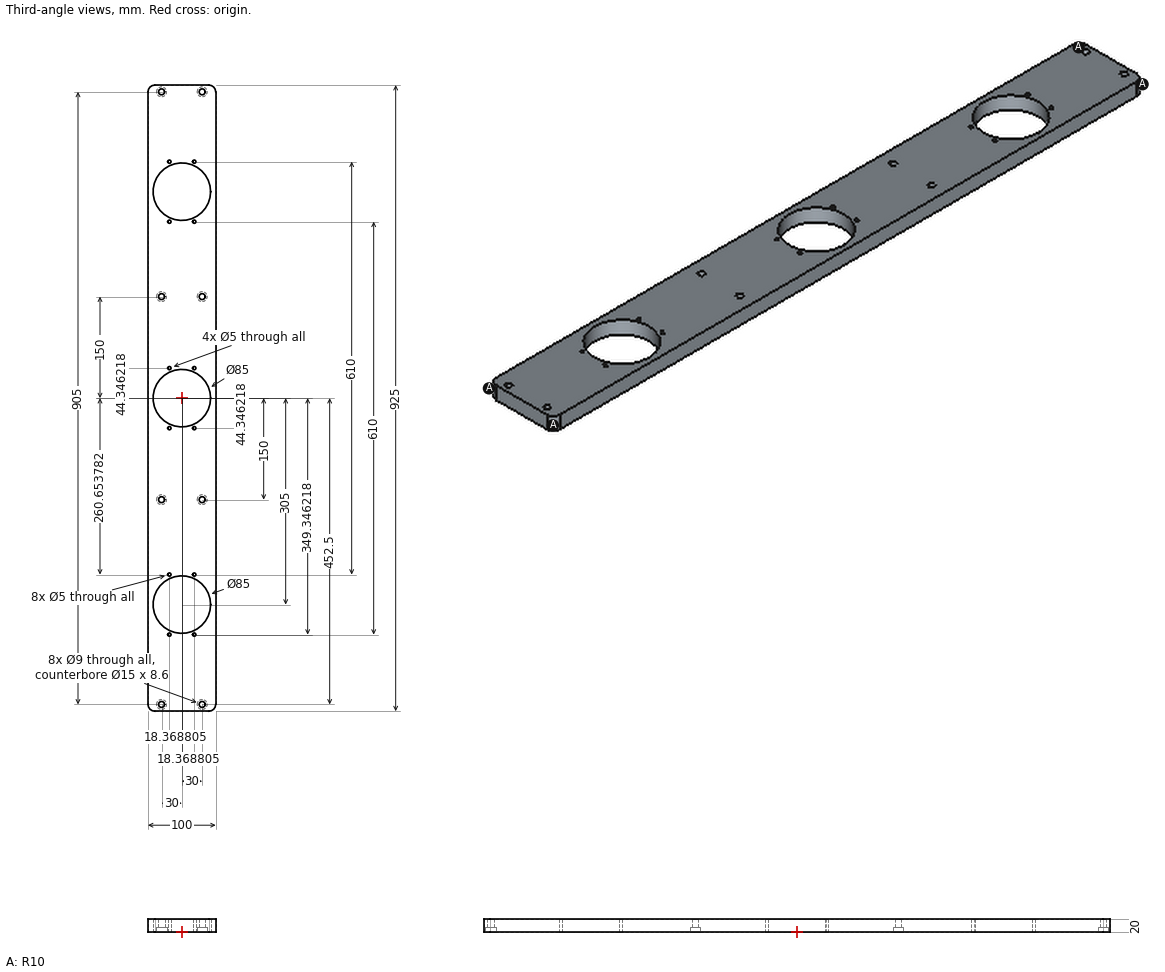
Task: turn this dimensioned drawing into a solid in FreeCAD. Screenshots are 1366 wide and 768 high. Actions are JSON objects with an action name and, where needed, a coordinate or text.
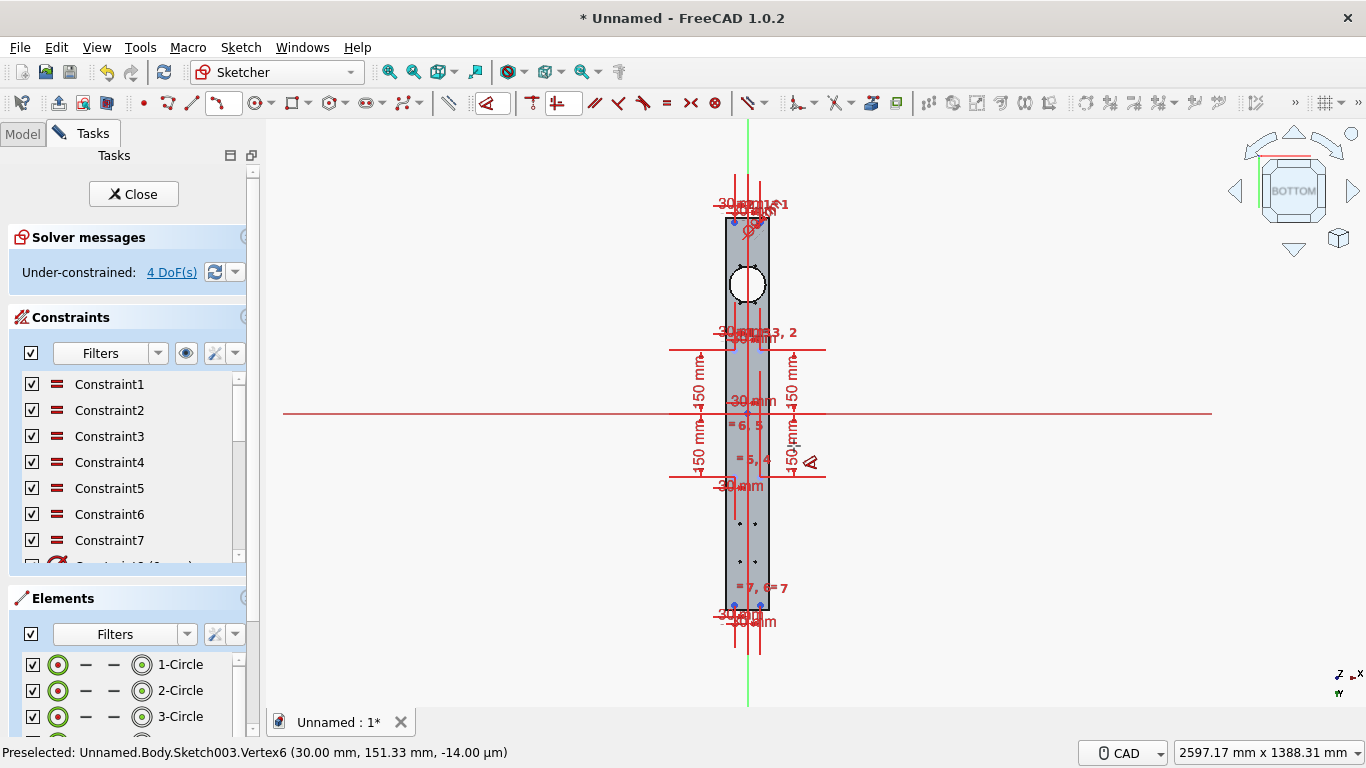
{"action": "left_click", "coordinate": [735, 223]}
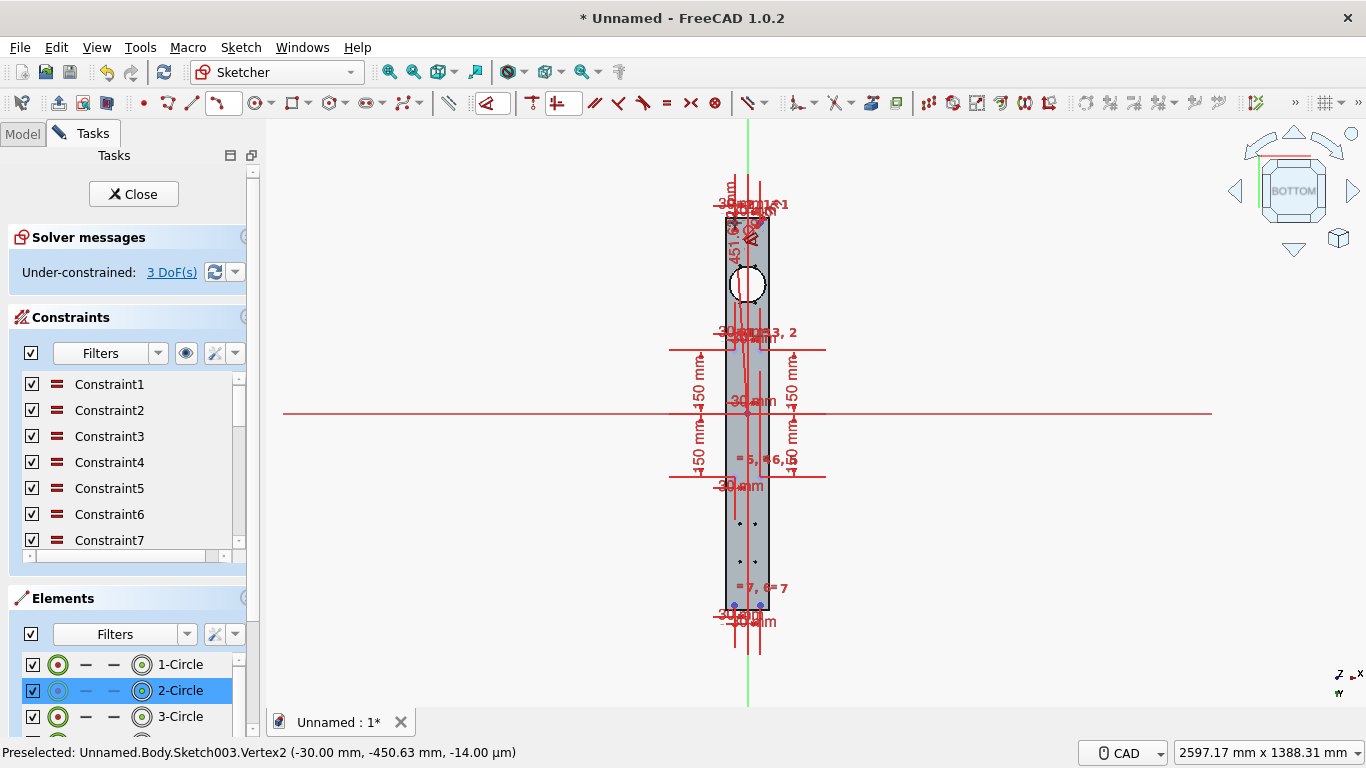
{"action": "left_click", "coordinate": [735, 606]}
{"action": "left_click", "coordinate": [701, 280]}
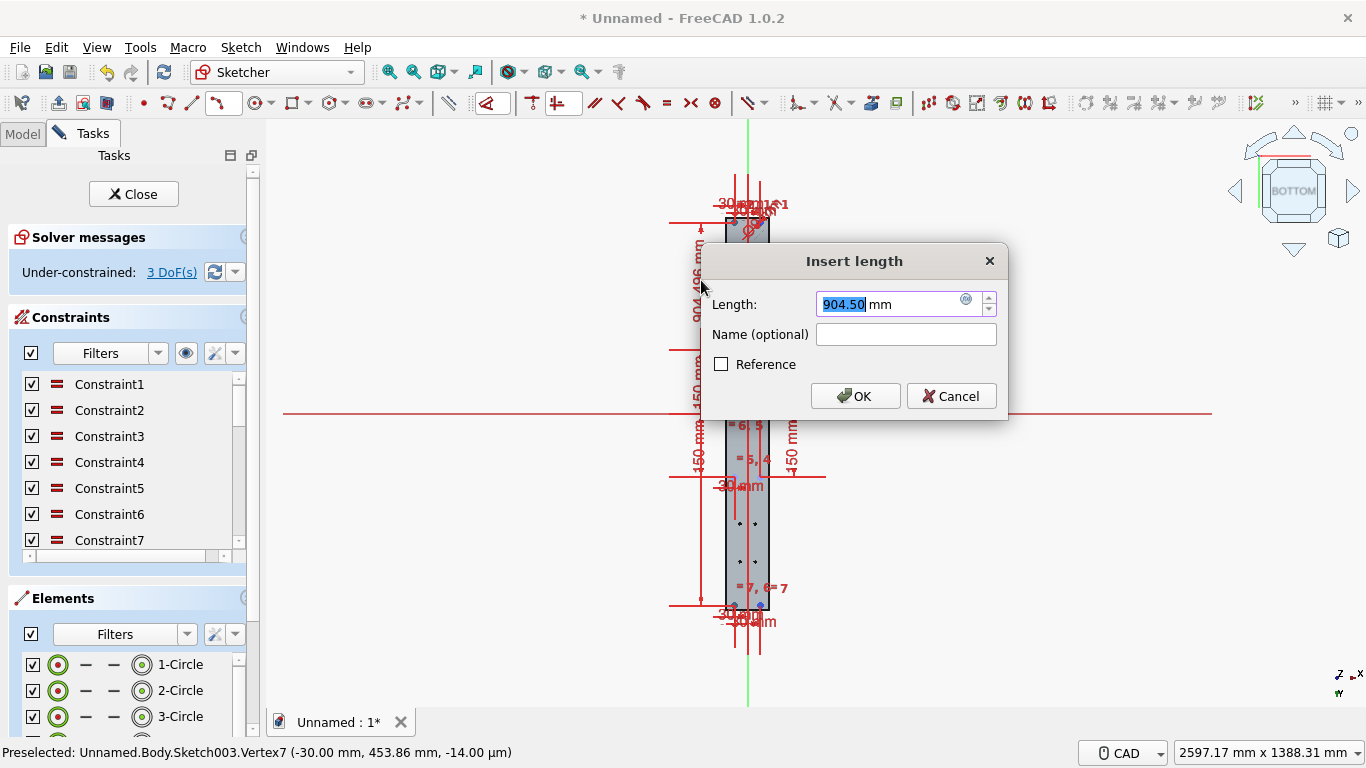
{"action": "type", "text": "905"}
{"action": "key", "text": "Return"}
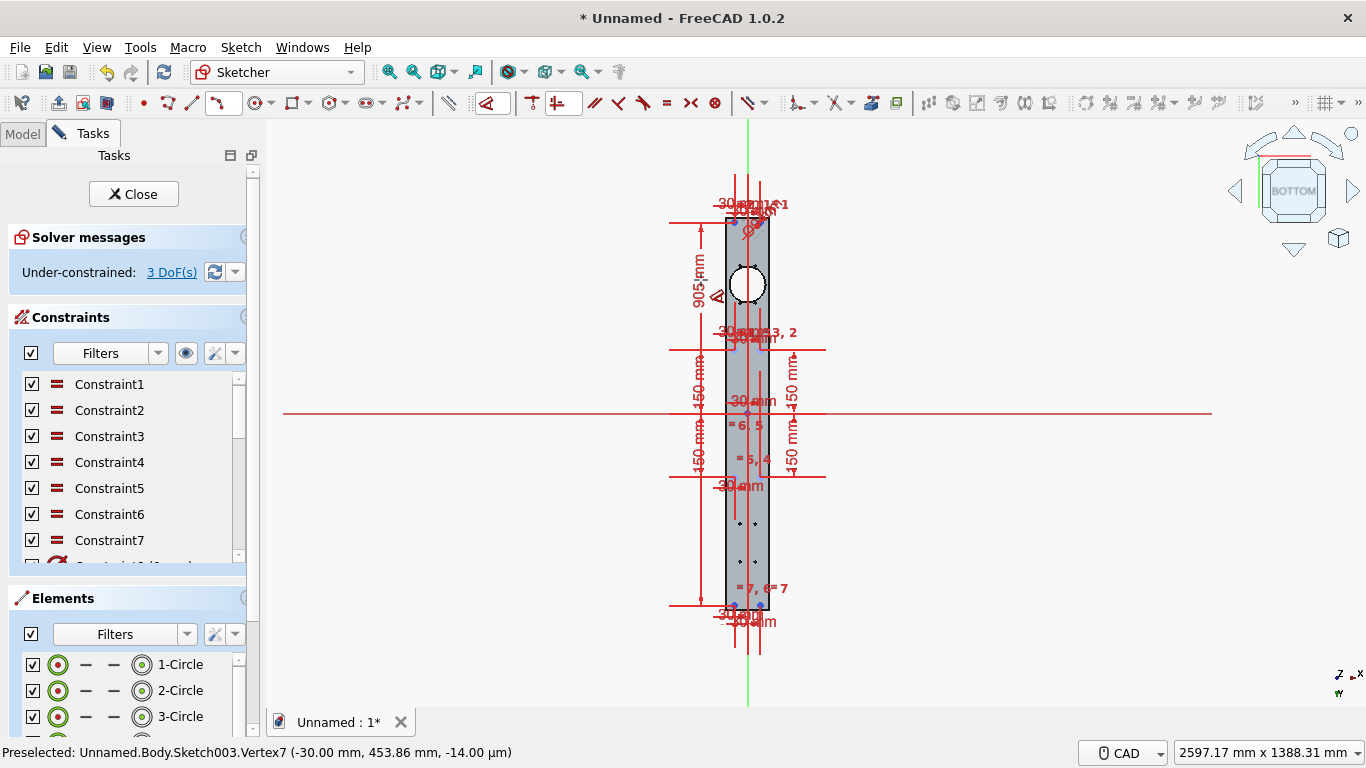
{"action": "left_click", "coordinate": [760, 223]}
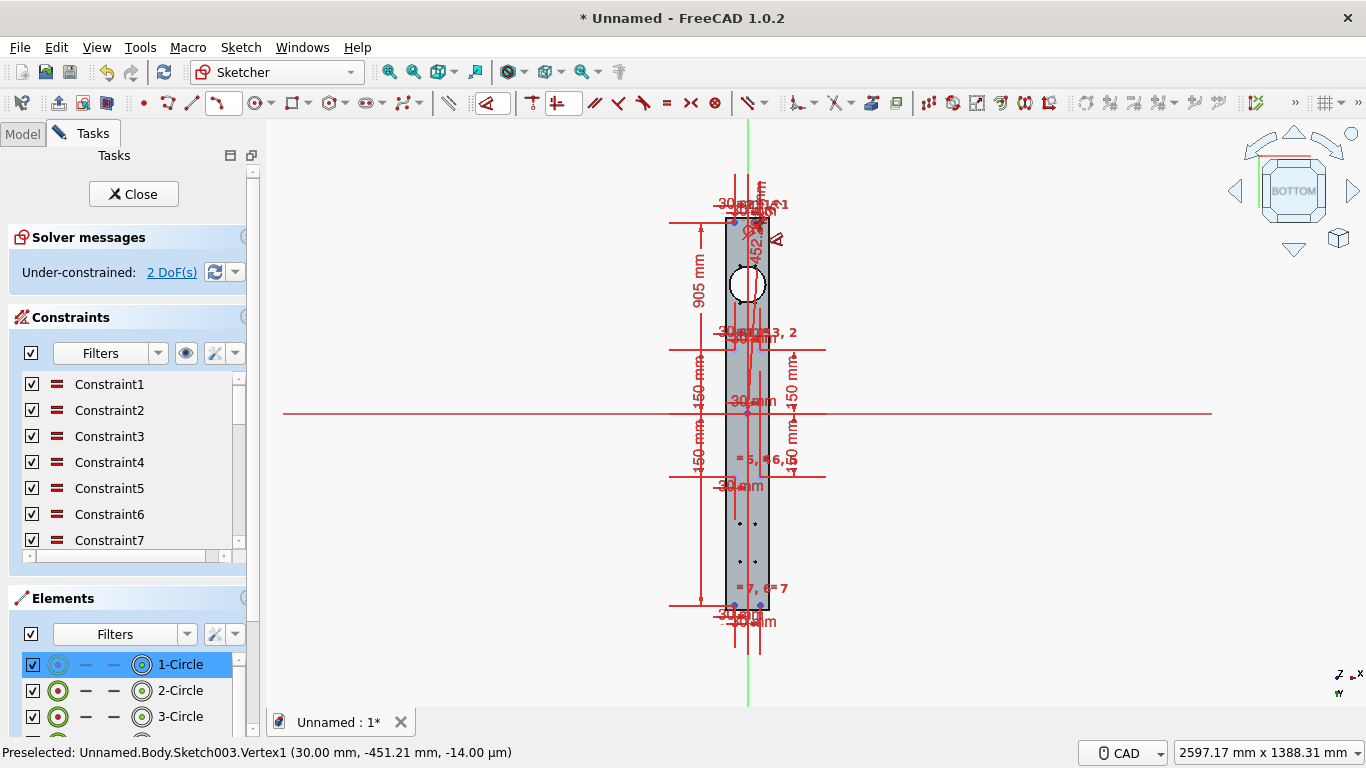
{"action": "left_click", "coordinate": [735, 606]}
{"action": "left_click", "coordinate": [794, 280]}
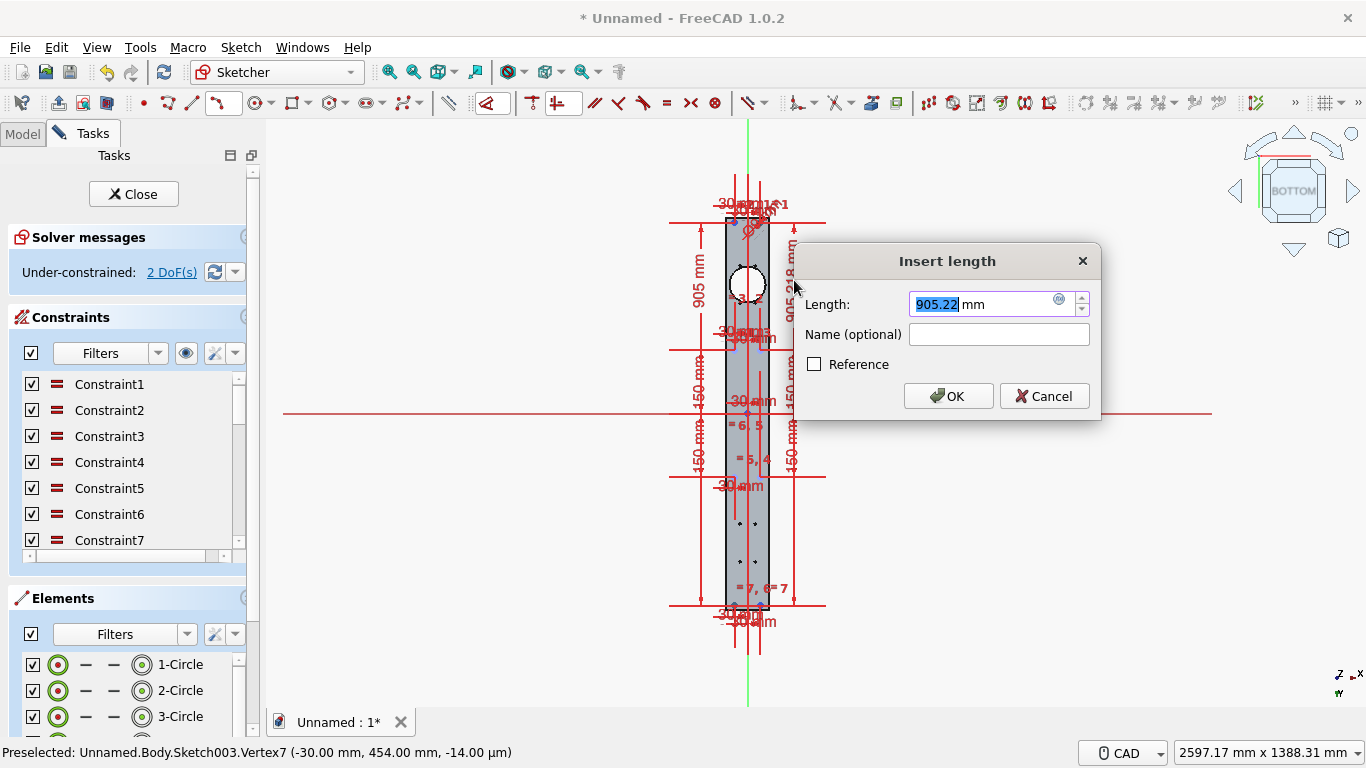
{"action": "type", "text": "905"}
{"action": "key", "text": "Return"}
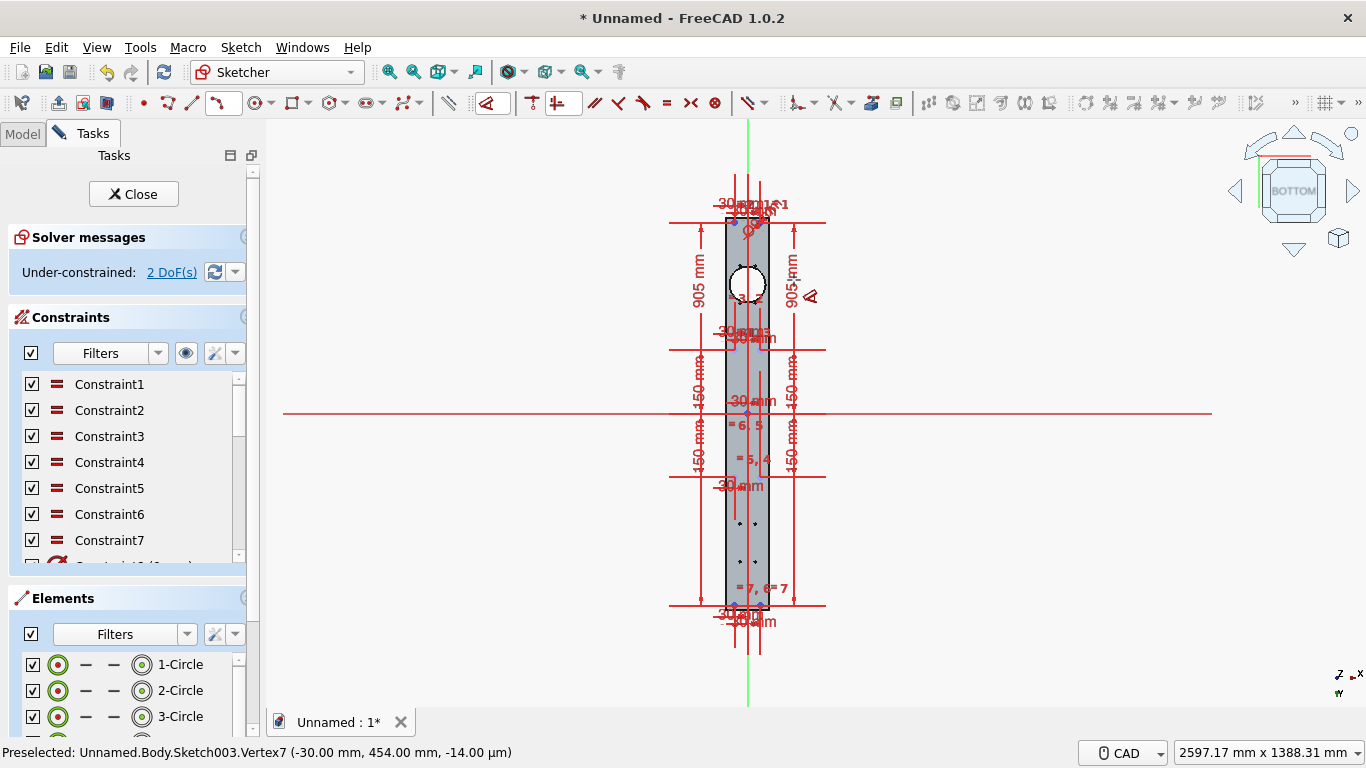
{"action": "left_click", "coordinate": [760, 223]}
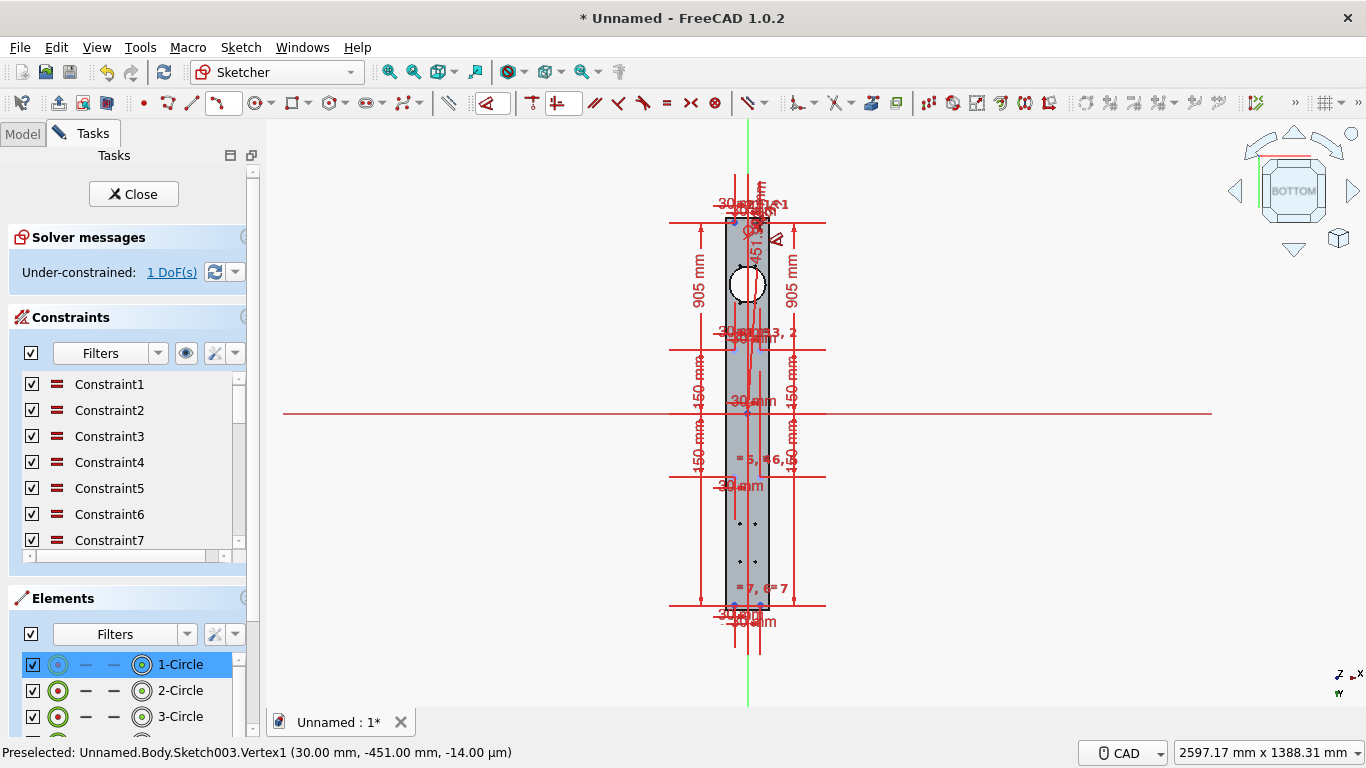
{"action": "left_click", "coordinate": [760, 606]}
{"action": "left_click", "coordinate": [794, 548]}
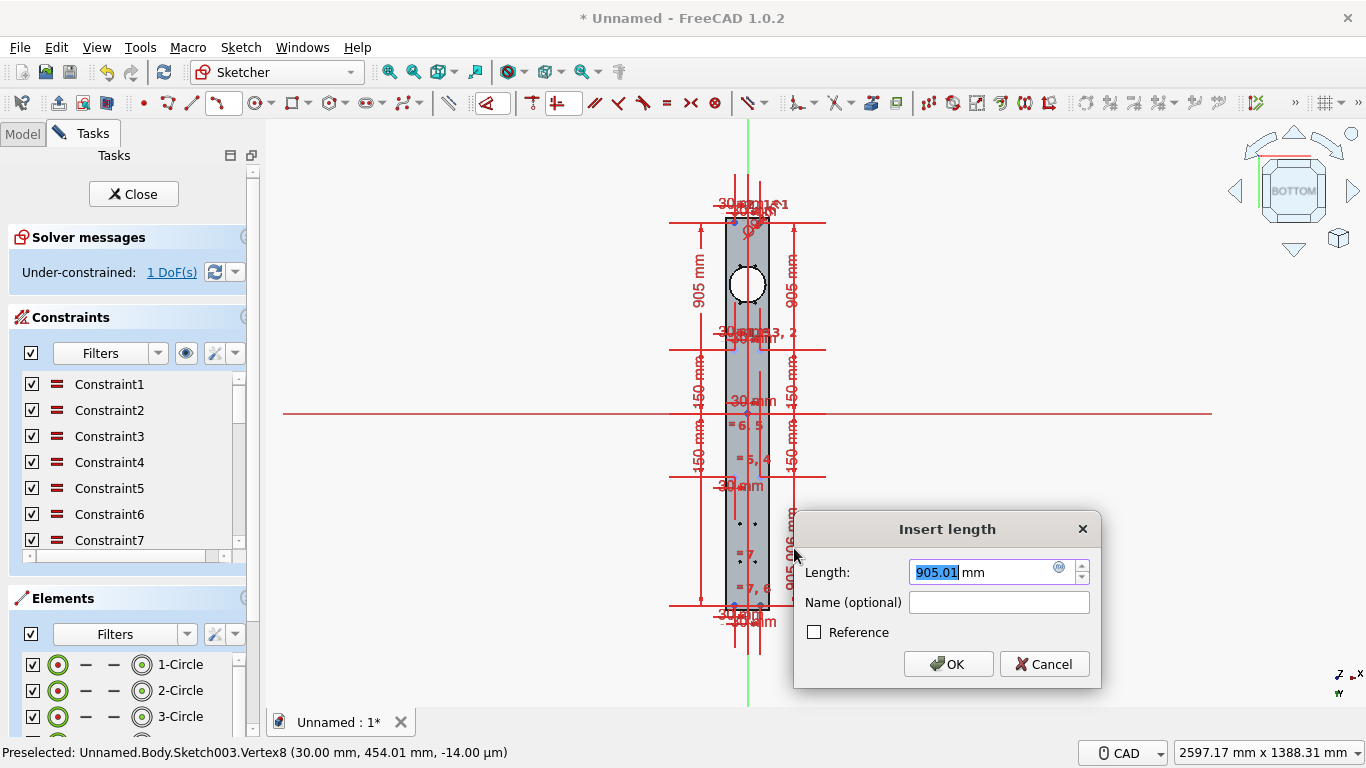
{"action": "type", "text": "905"}
{"action": "key", "text": "Return"}